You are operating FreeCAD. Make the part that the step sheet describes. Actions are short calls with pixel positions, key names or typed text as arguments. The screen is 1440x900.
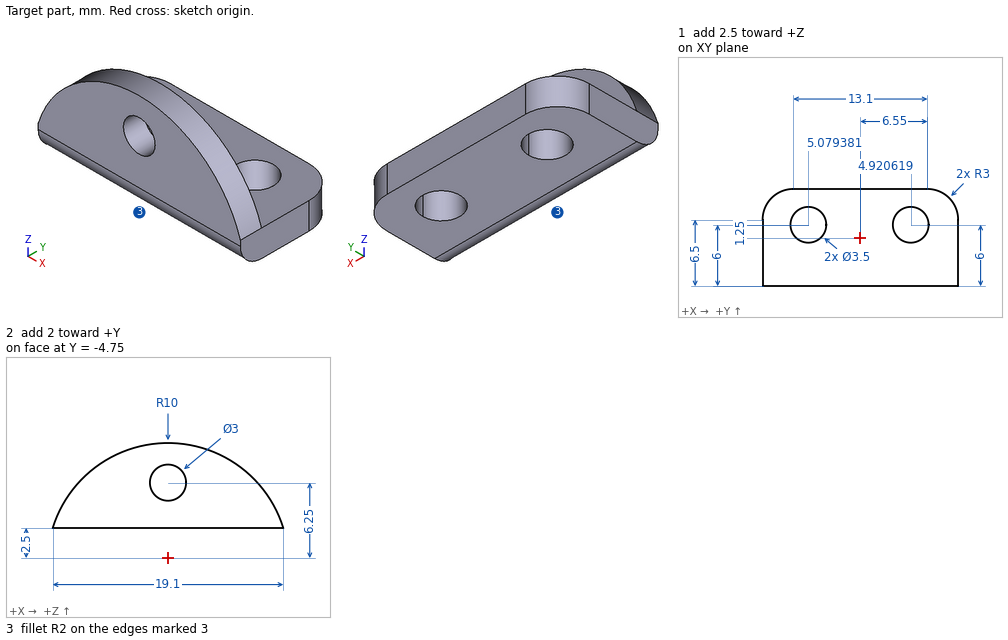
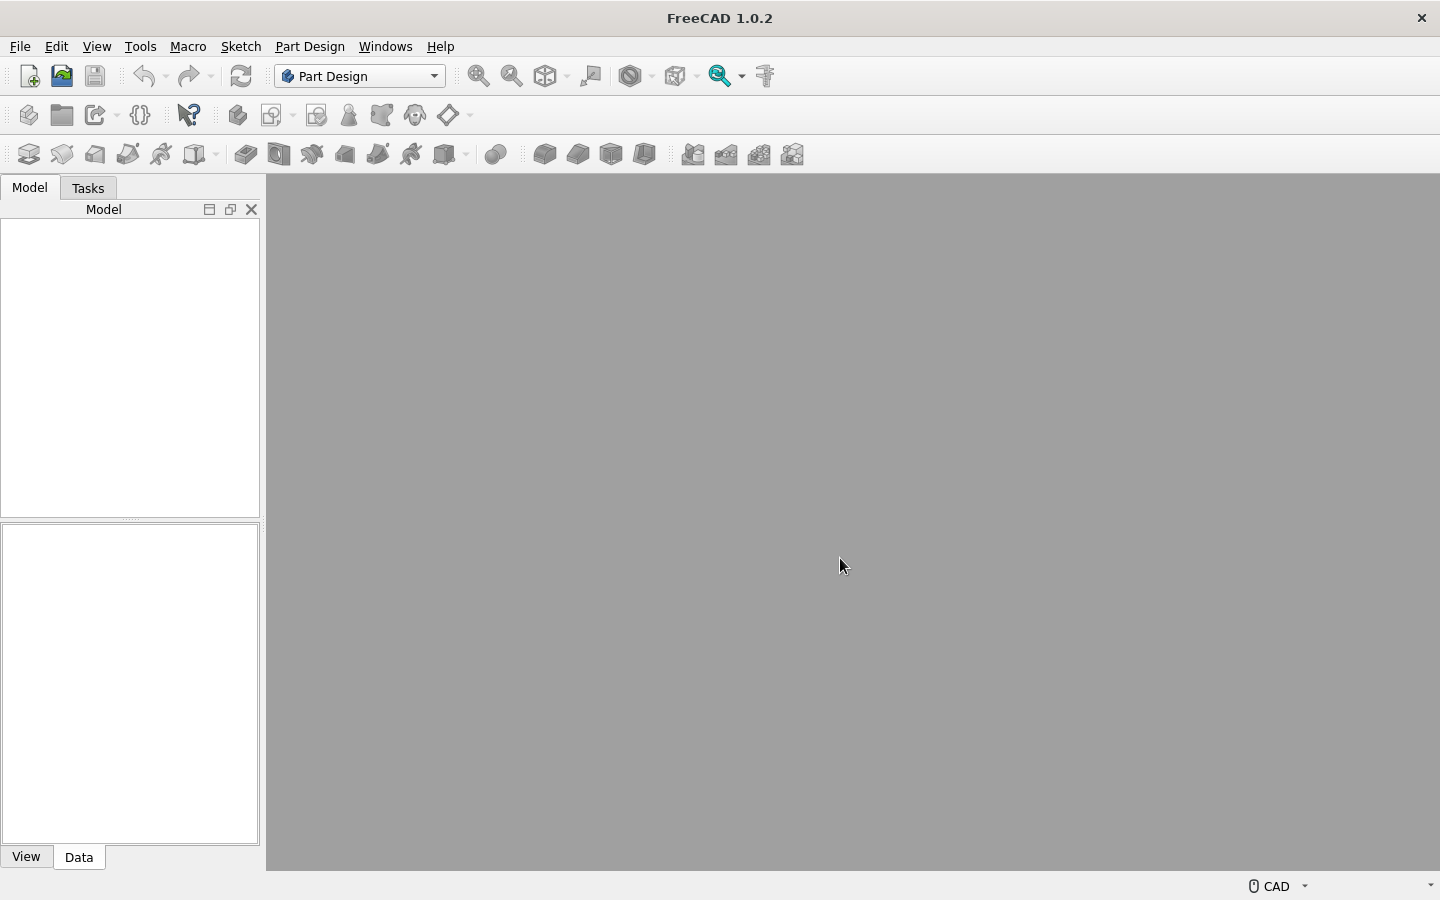
click(29, 76)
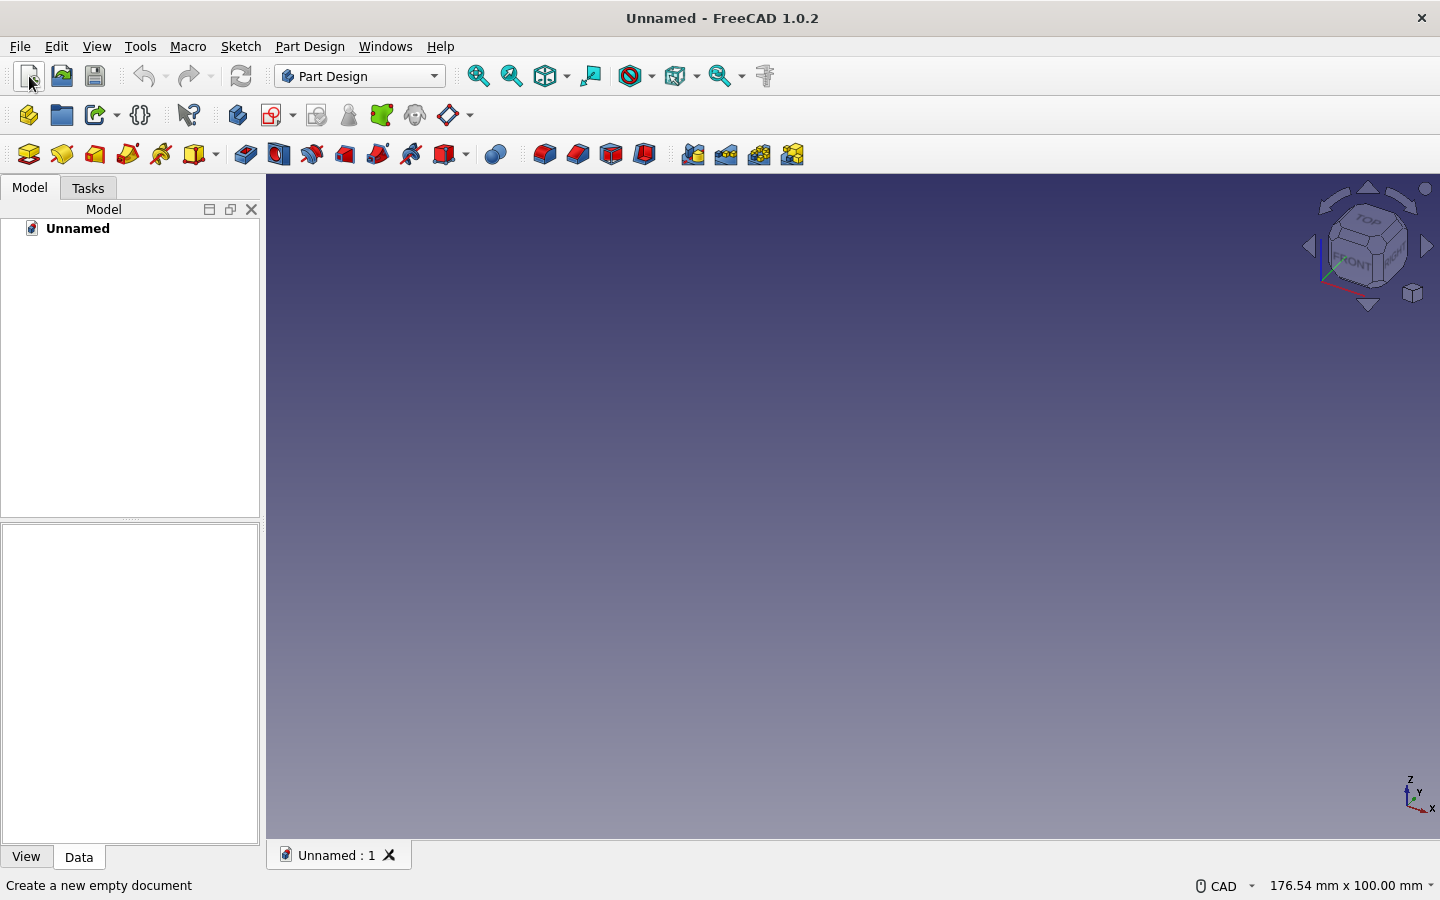
click(270, 116)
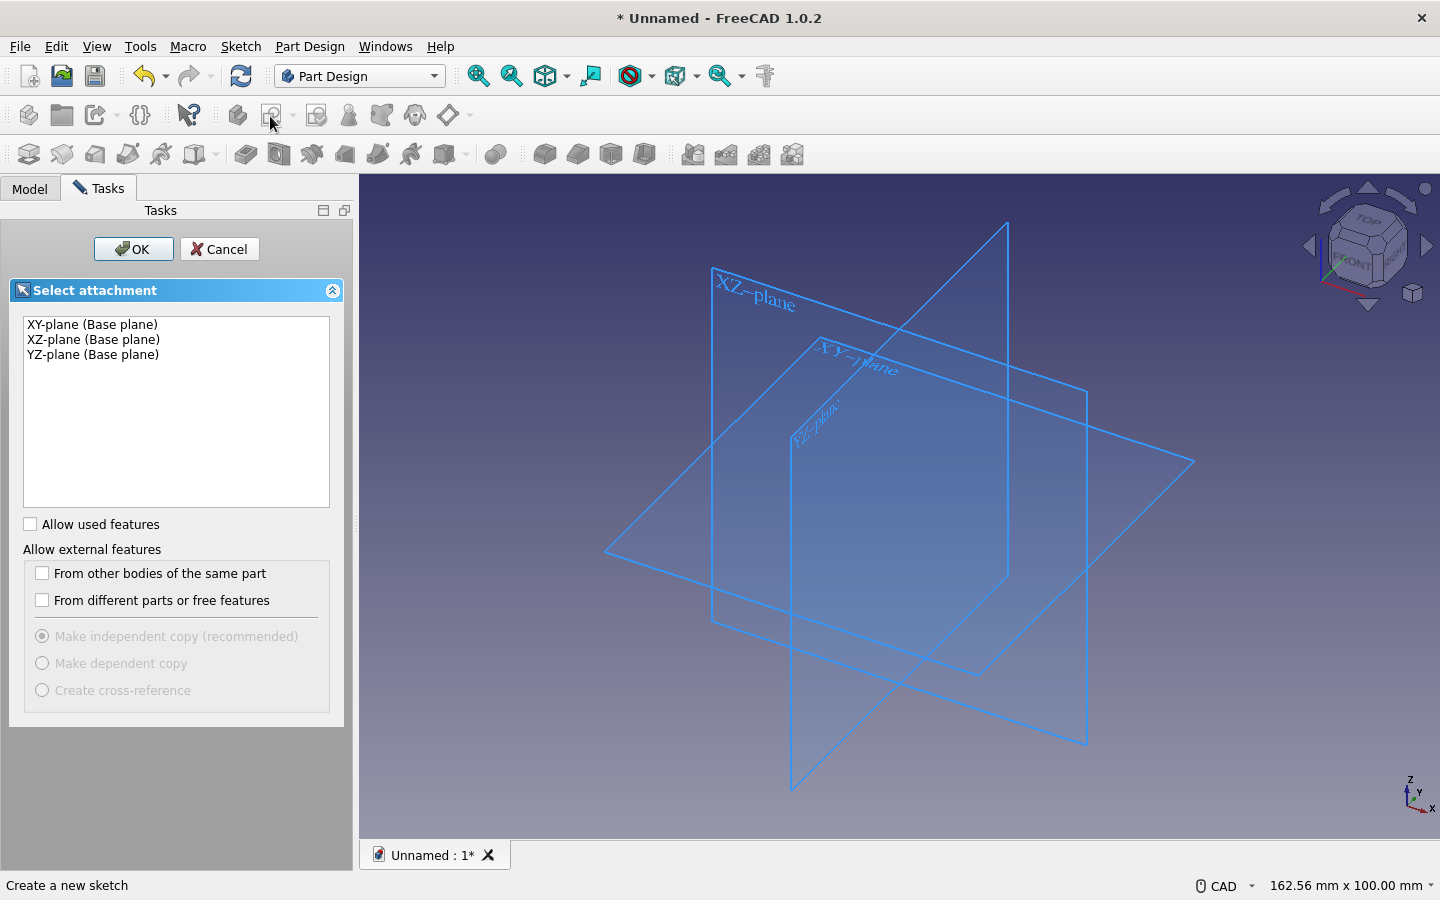
click(84, 324)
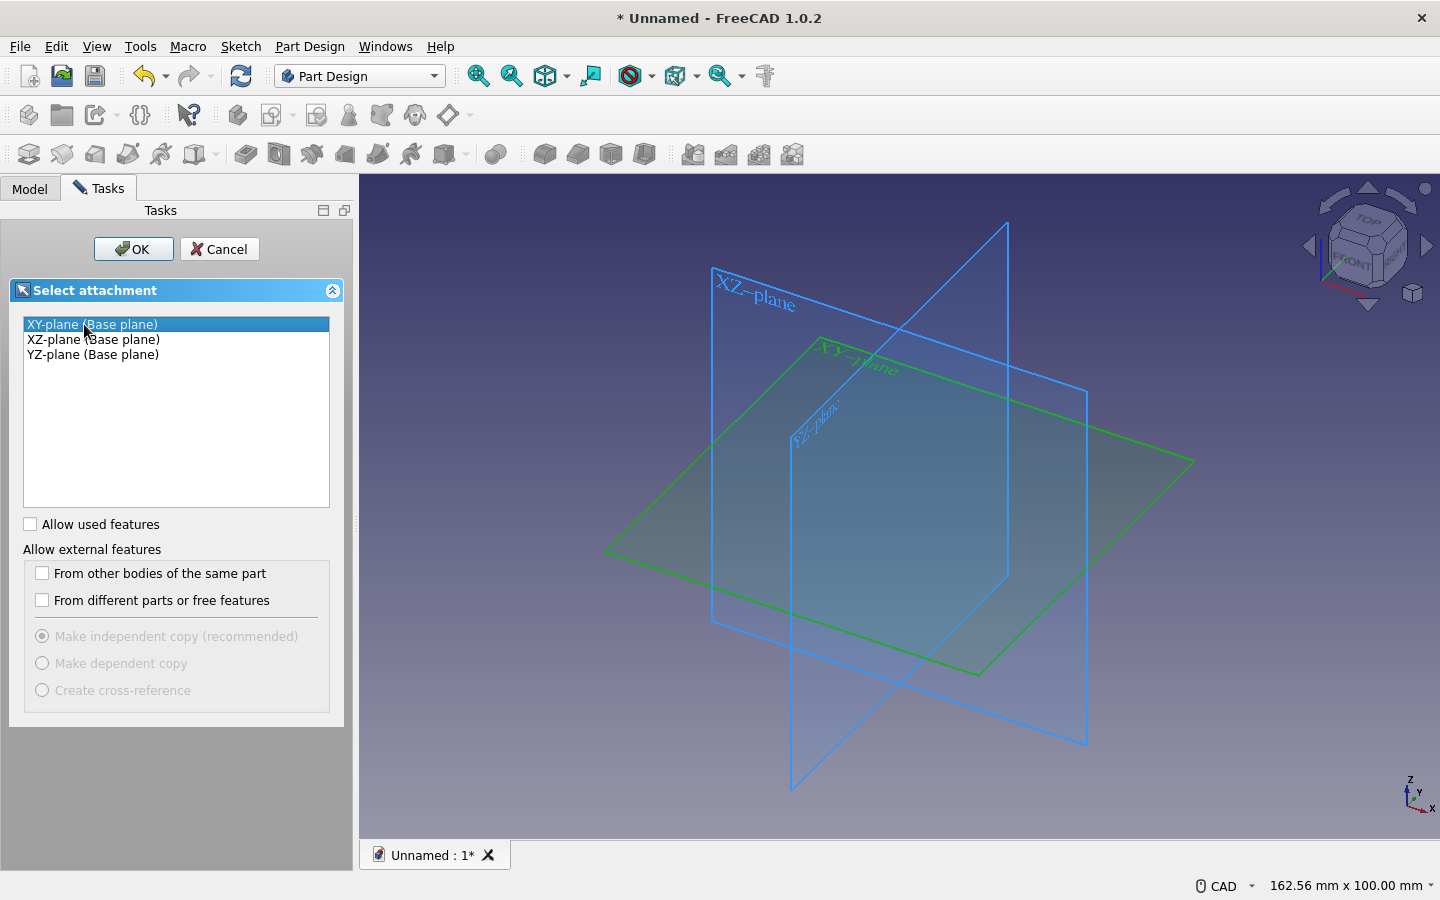
click(134, 249)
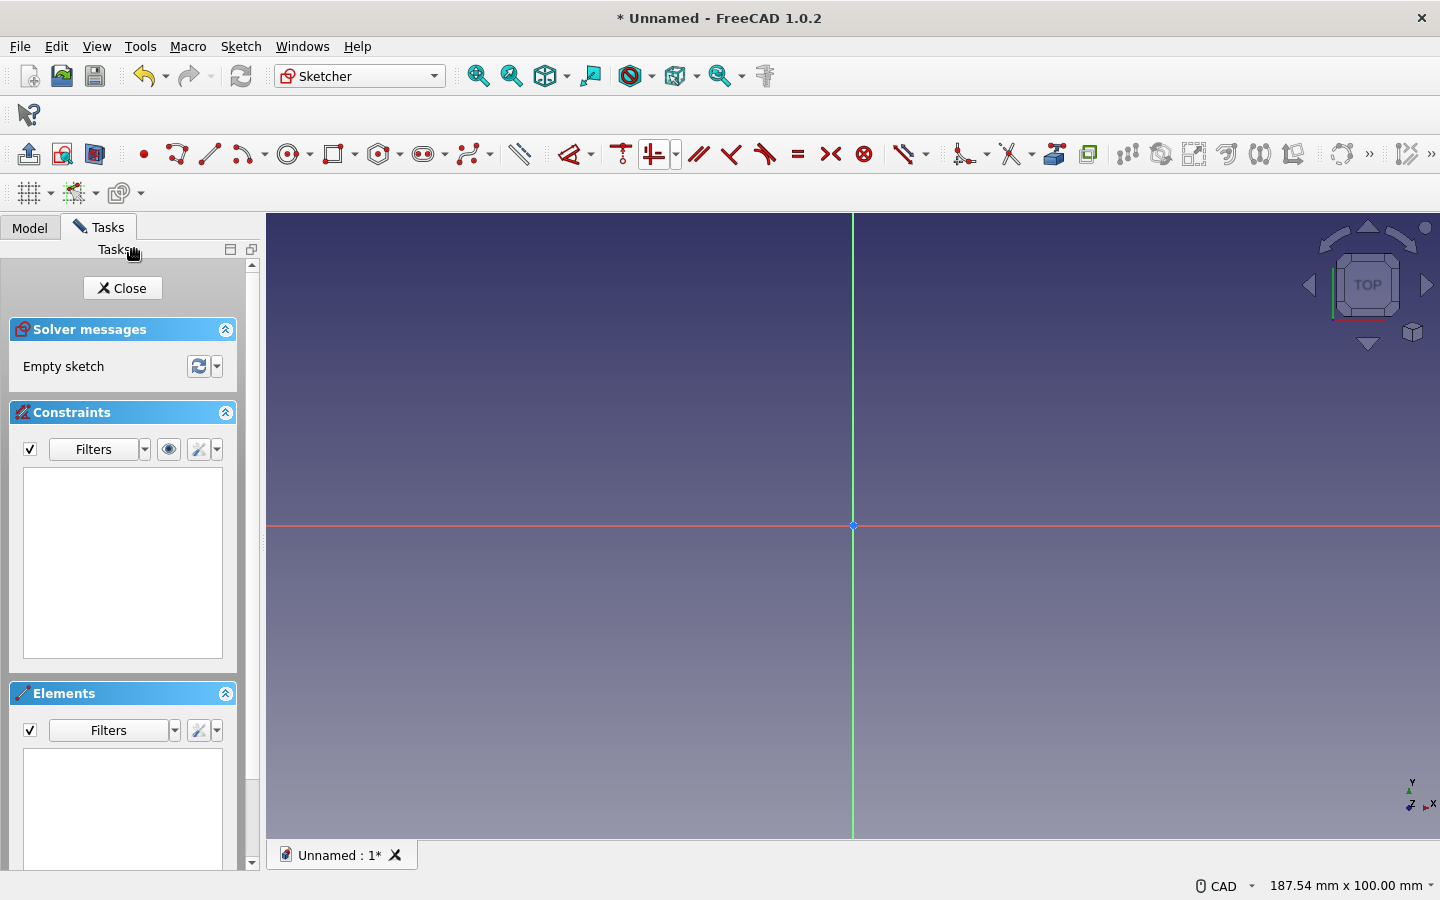
scroll(867, 526, up, 9)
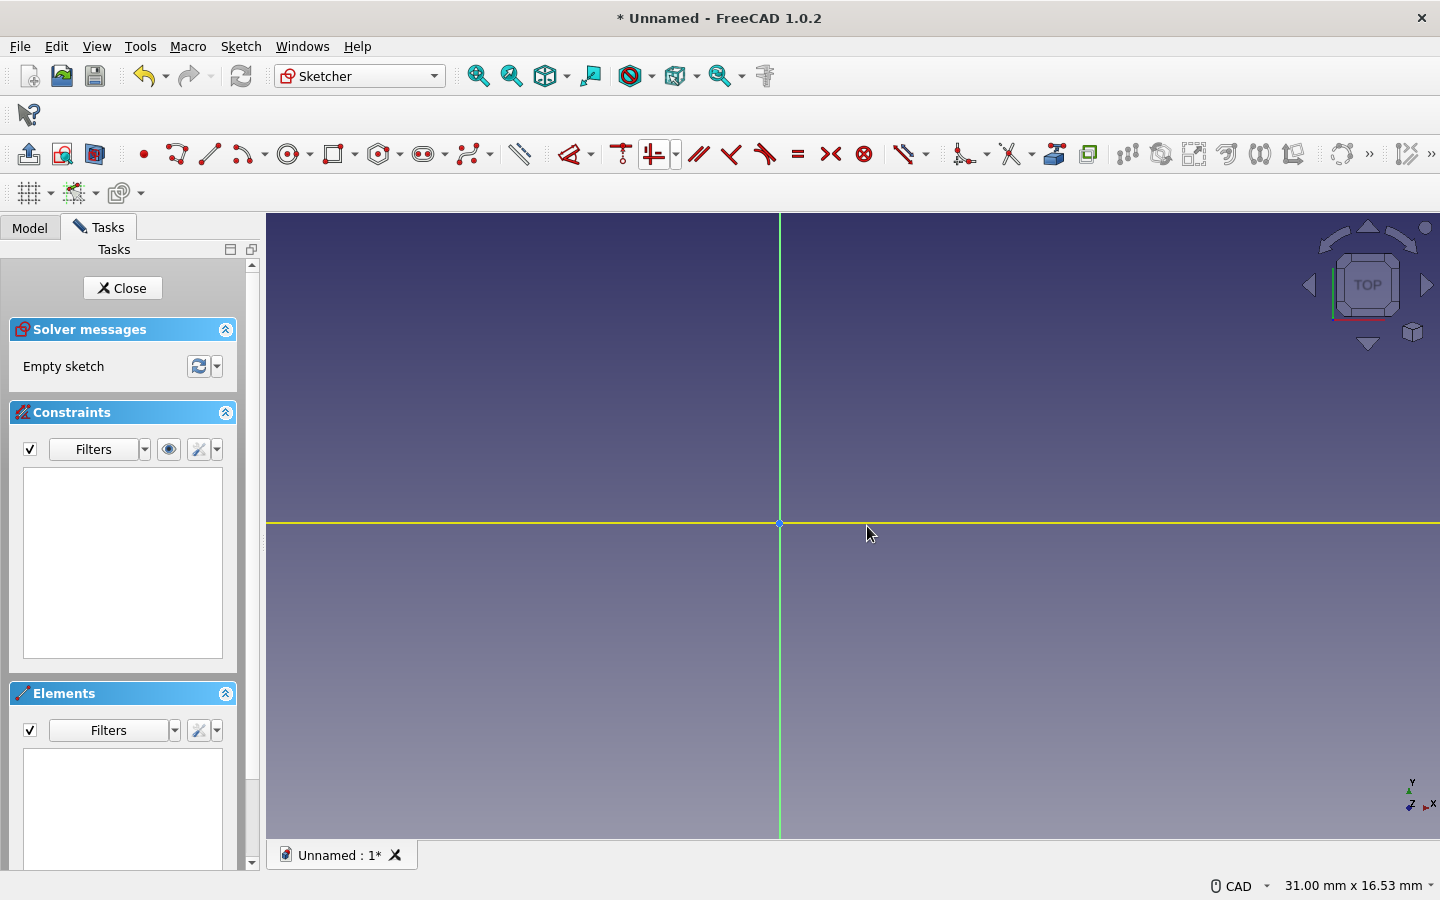
click(210, 154)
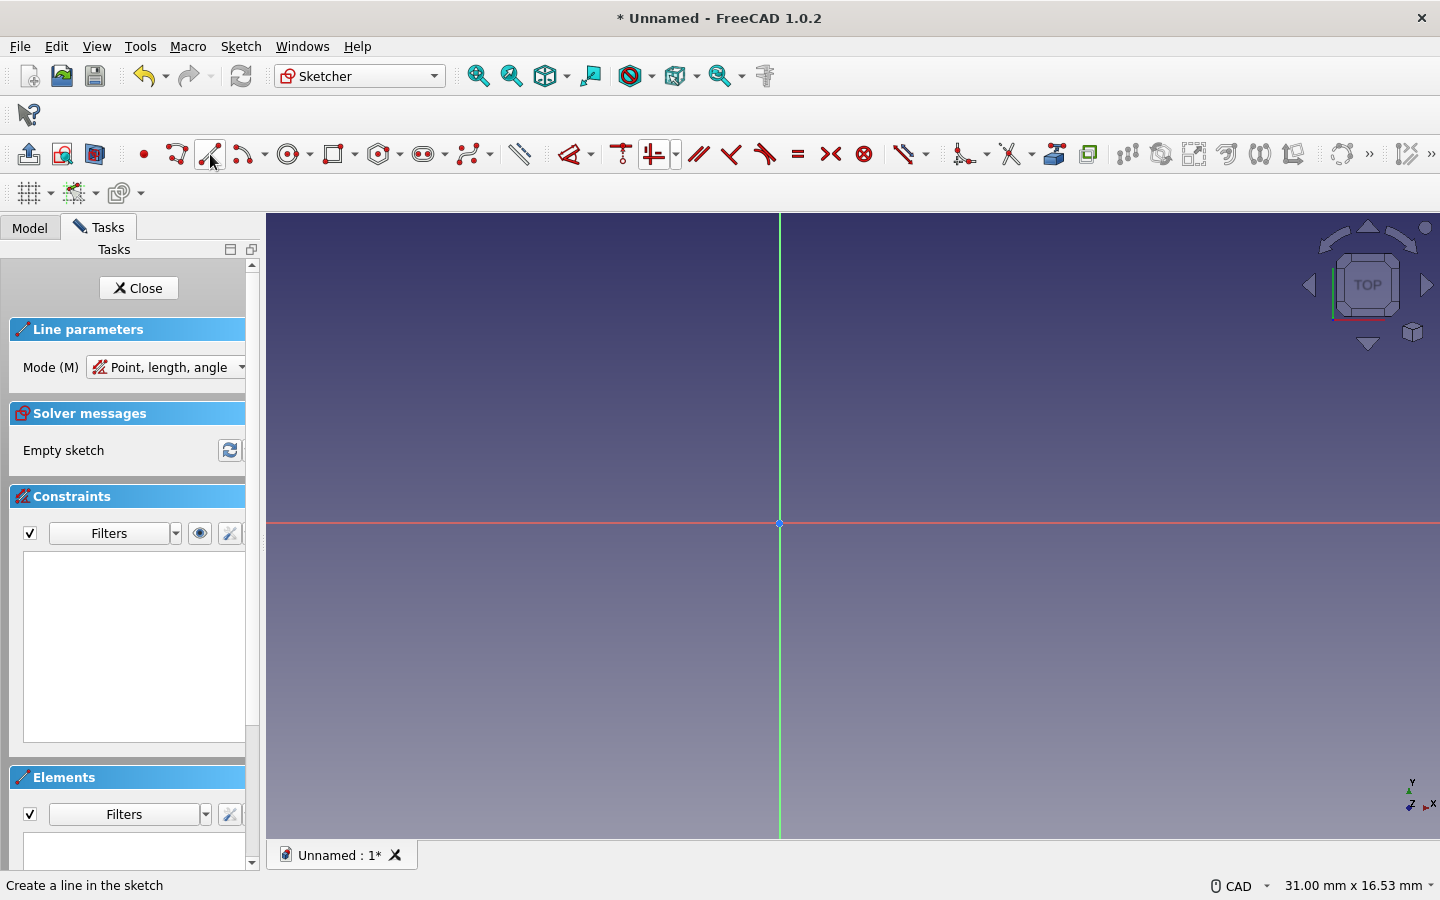
click(1028, 344)
click(532, 344)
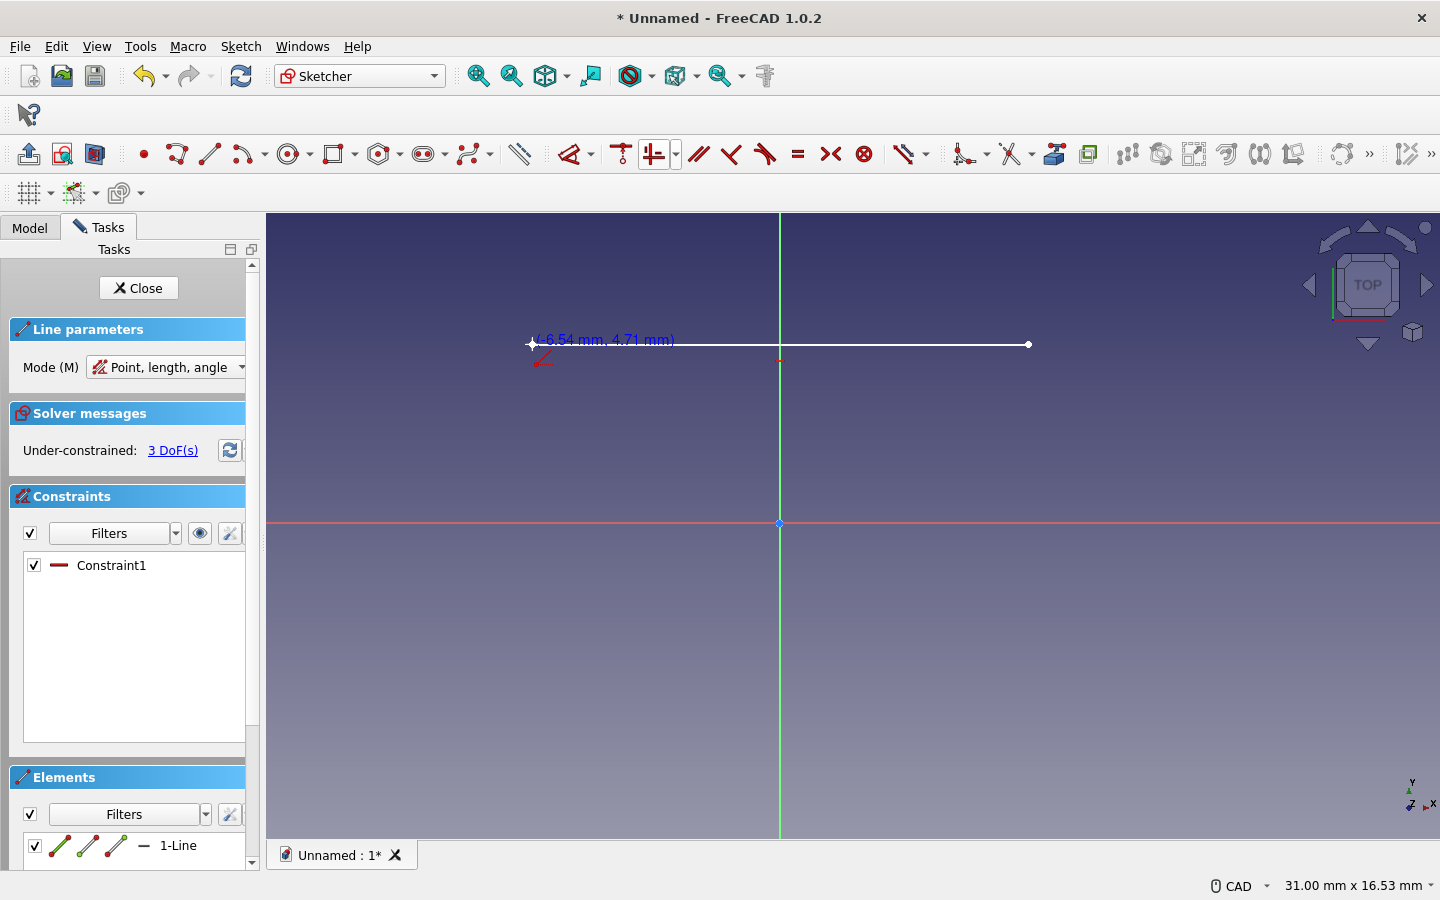
click(177, 154)